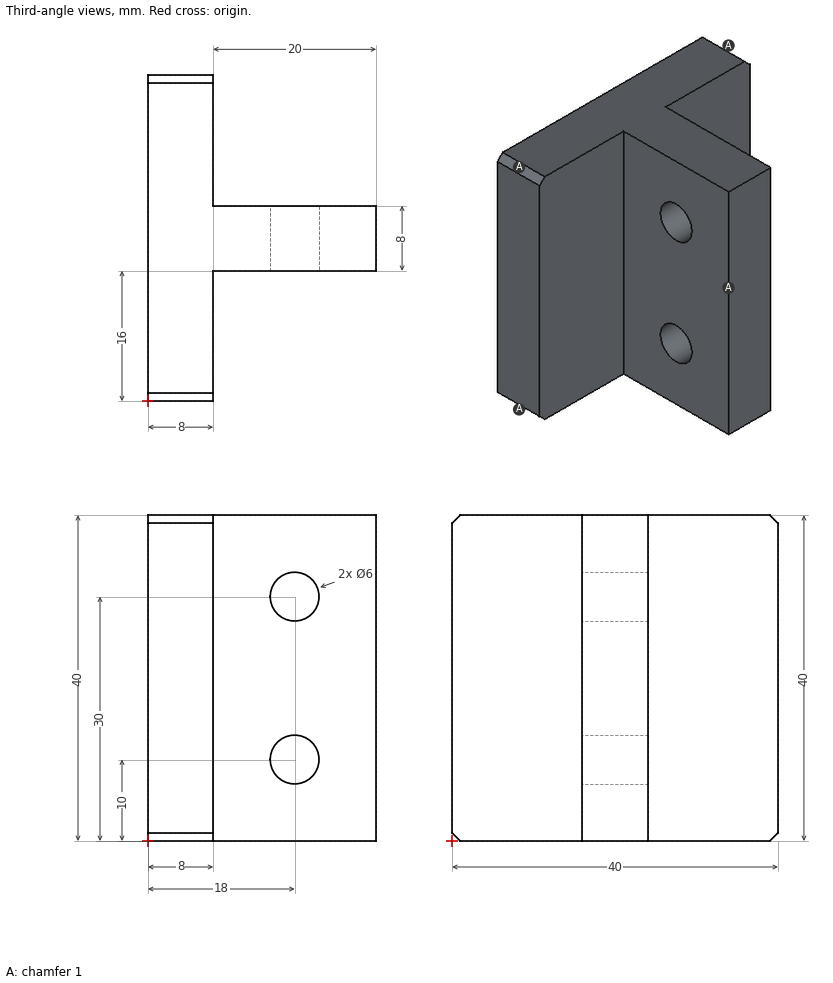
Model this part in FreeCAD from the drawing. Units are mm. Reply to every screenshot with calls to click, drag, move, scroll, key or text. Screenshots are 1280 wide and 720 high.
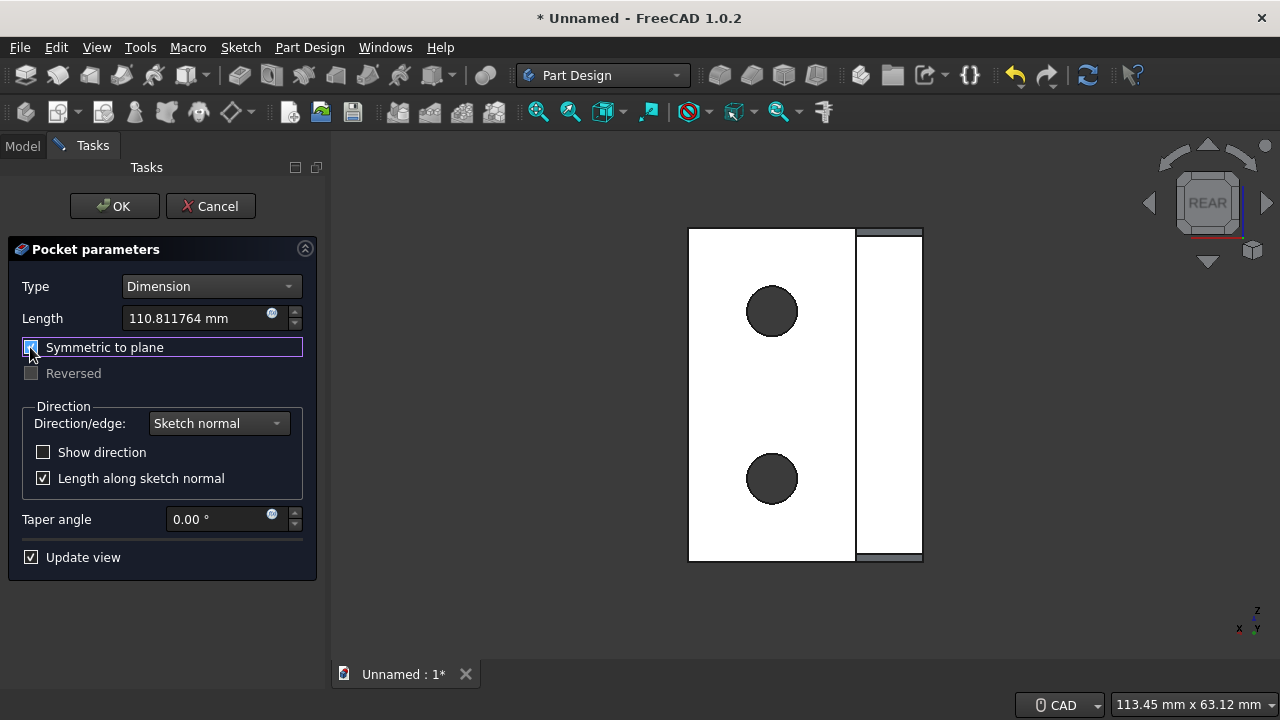
click(115, 206)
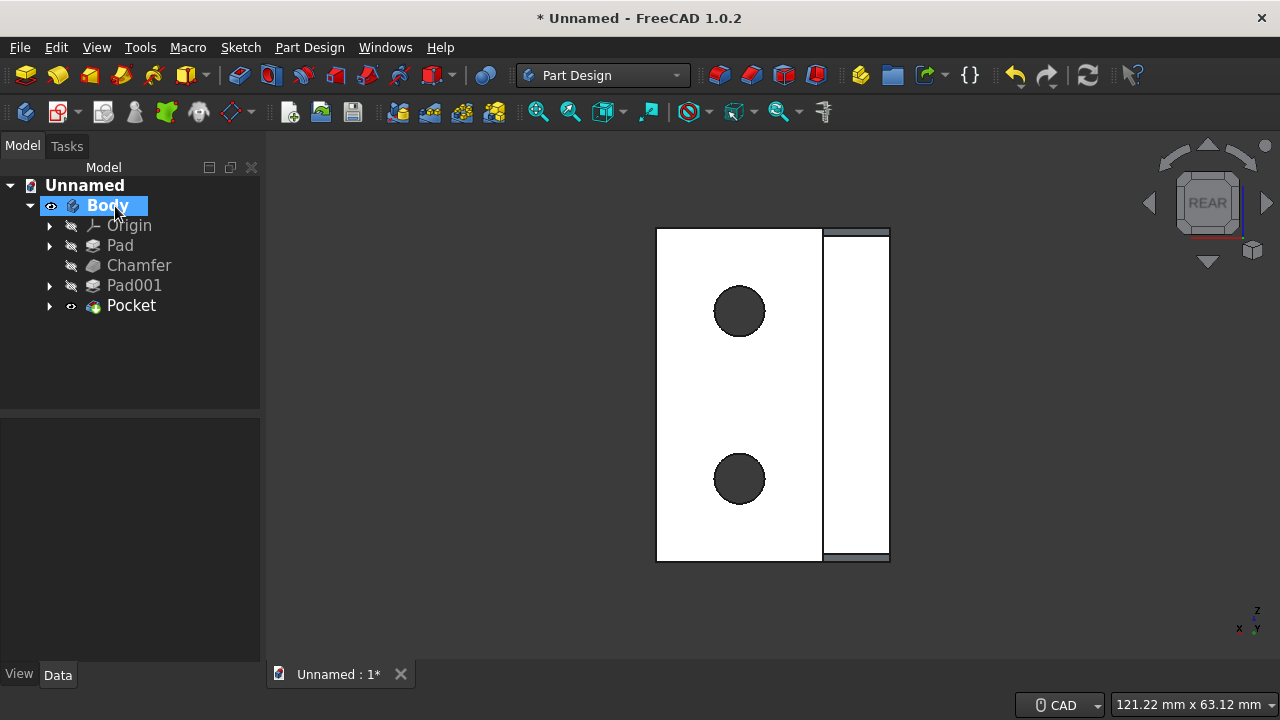
key(0)